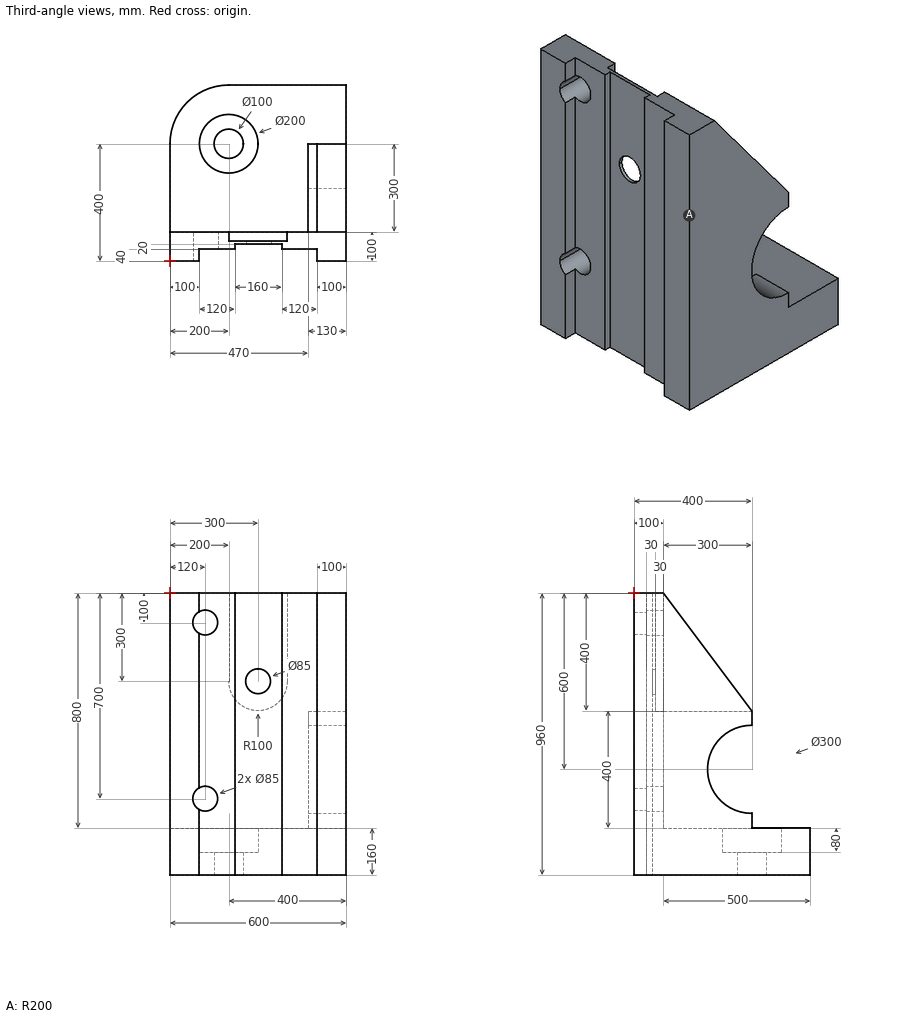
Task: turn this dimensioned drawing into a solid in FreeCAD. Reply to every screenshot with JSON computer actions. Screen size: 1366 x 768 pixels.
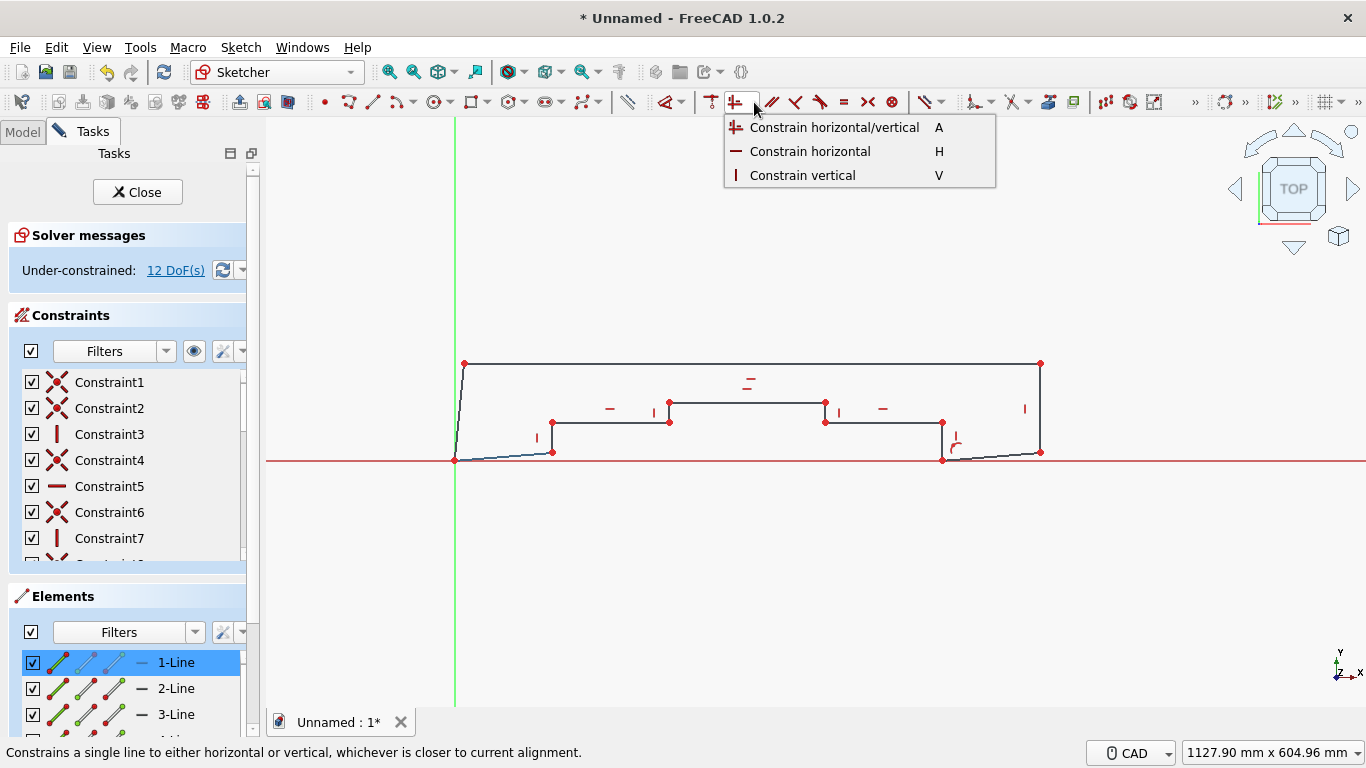
{"action": "left_click", "coordinate": [860, 151]}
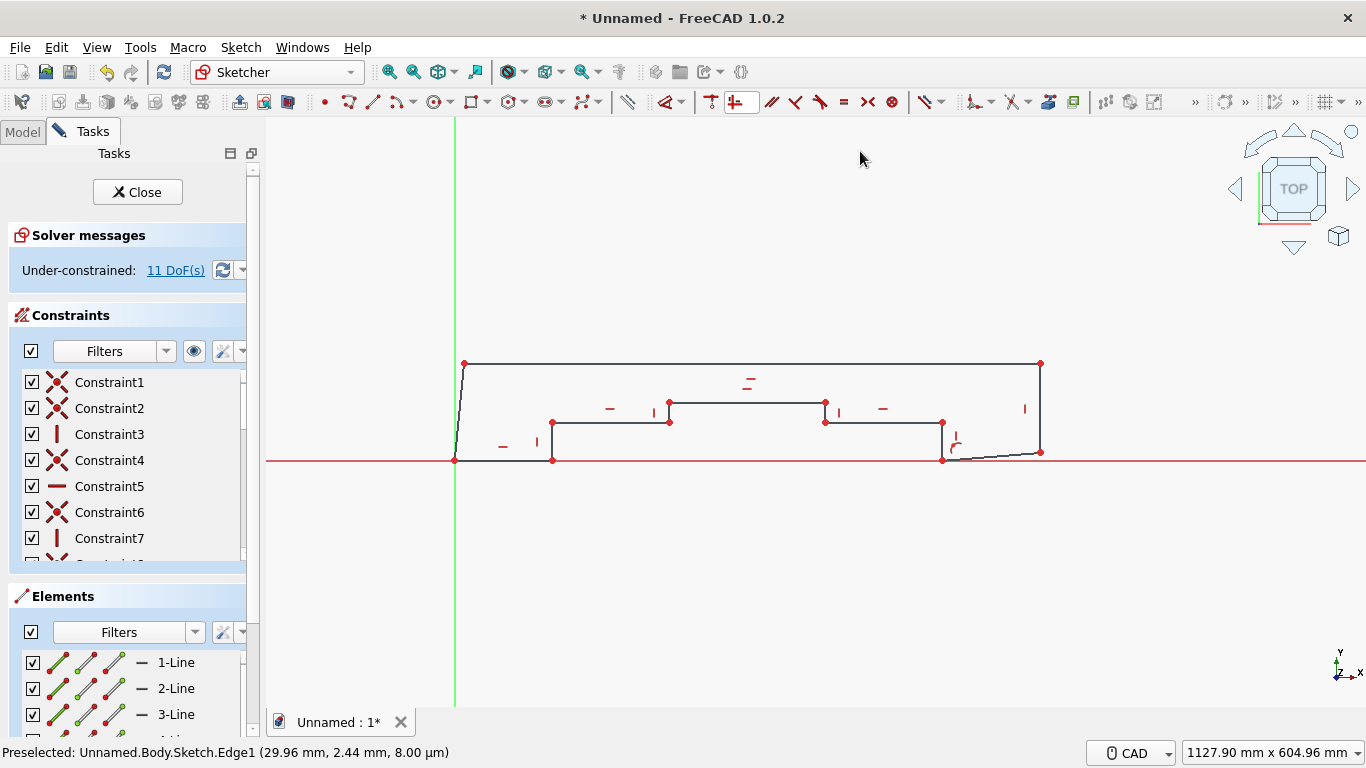
{"action": "left_click", "coordinate": [971, 459]}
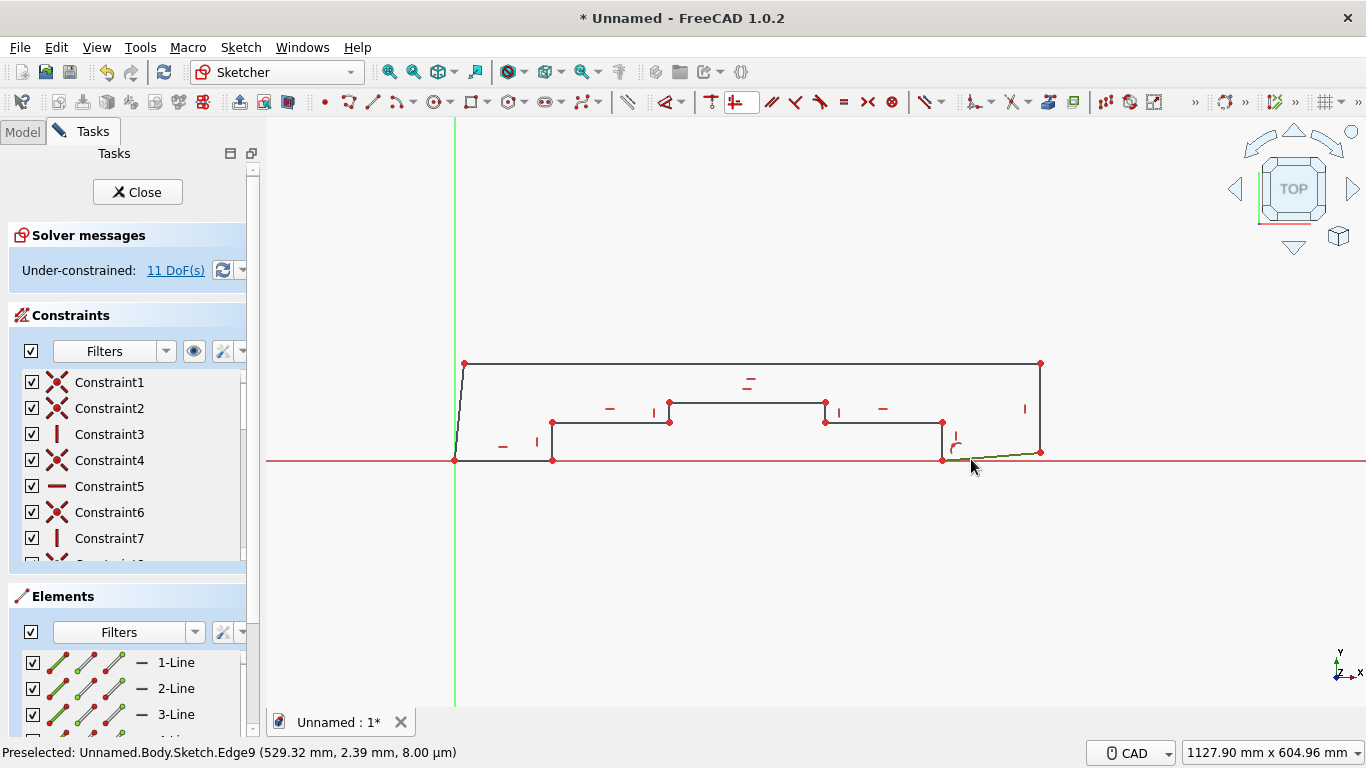
{"action": "key", "text": "h"}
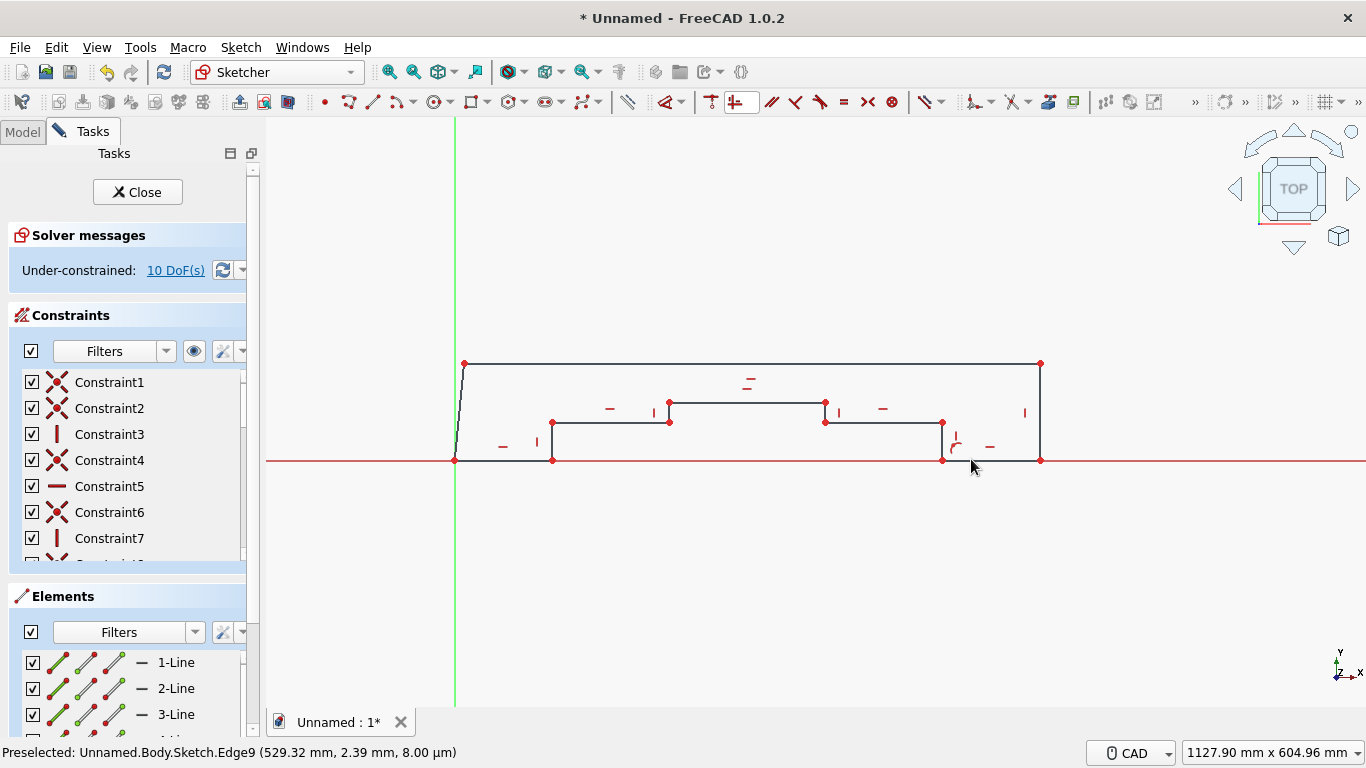
{"action": "left_click", "coordinate": [457, 432]}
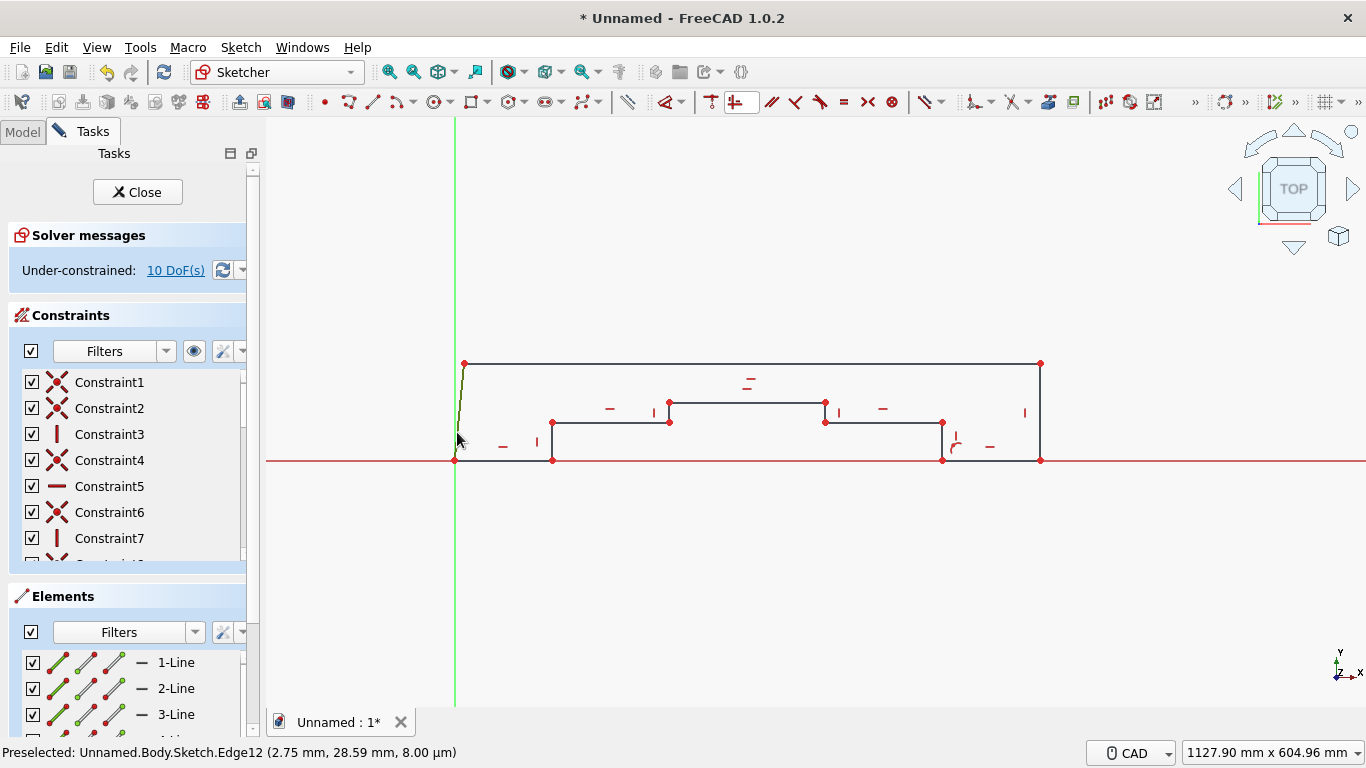
{"action": "key", "text": "v"}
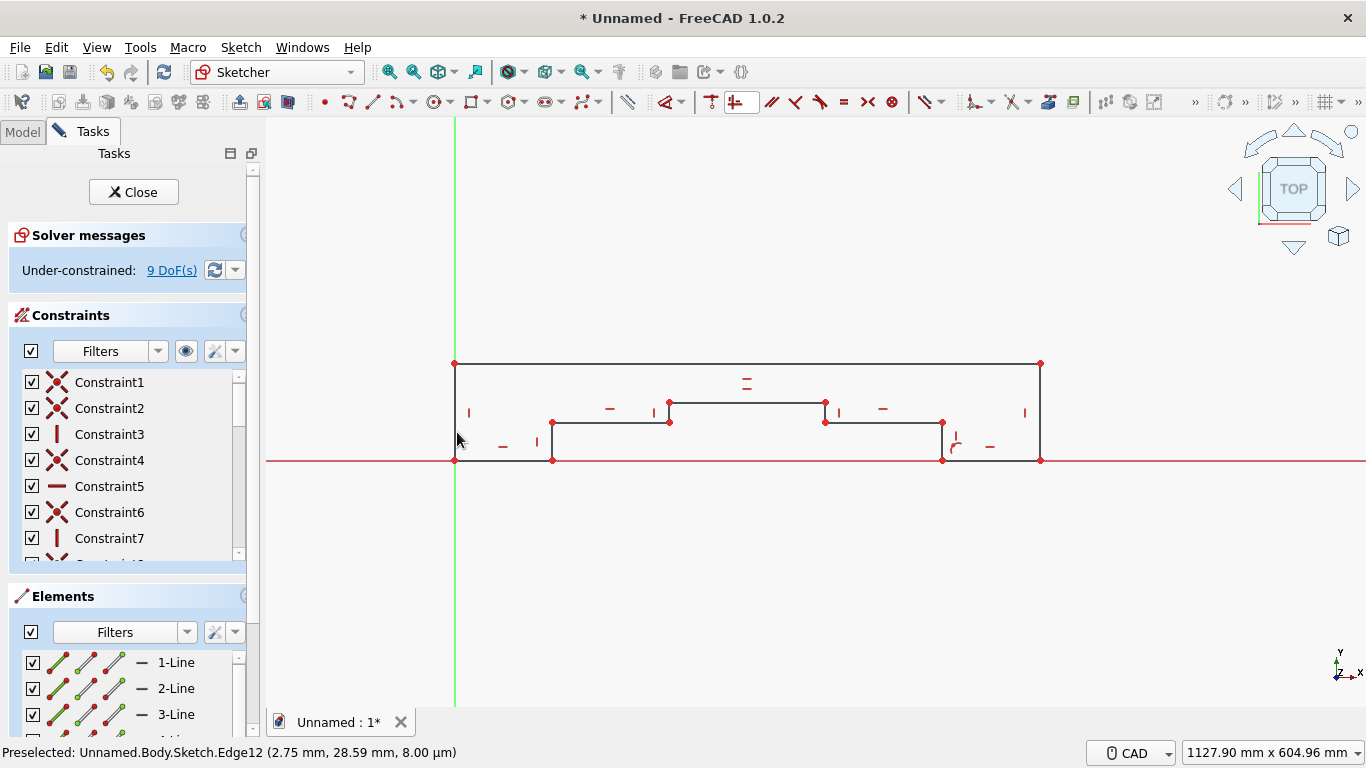
{"action": "left_click", "coordinate": [552, 450]}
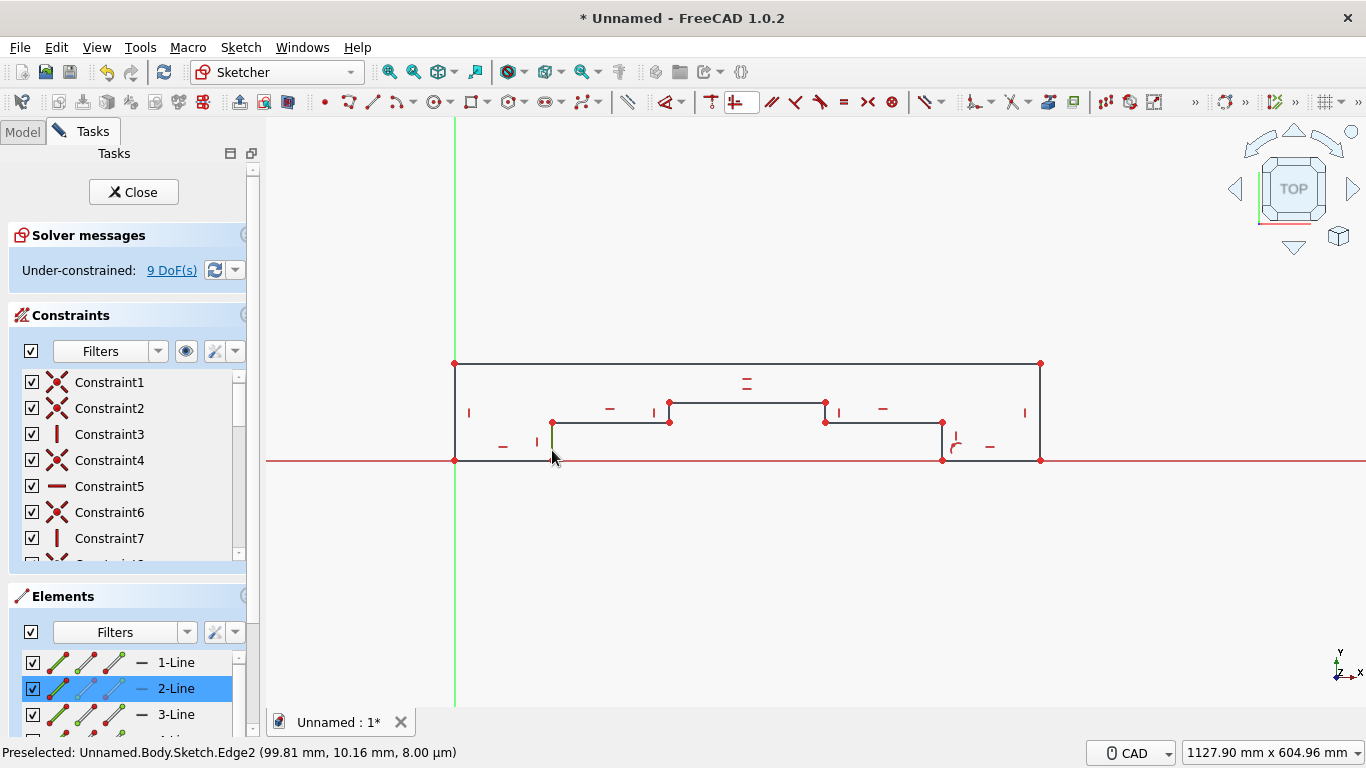
{"action": "left_click", "coordinate": [684, 102]}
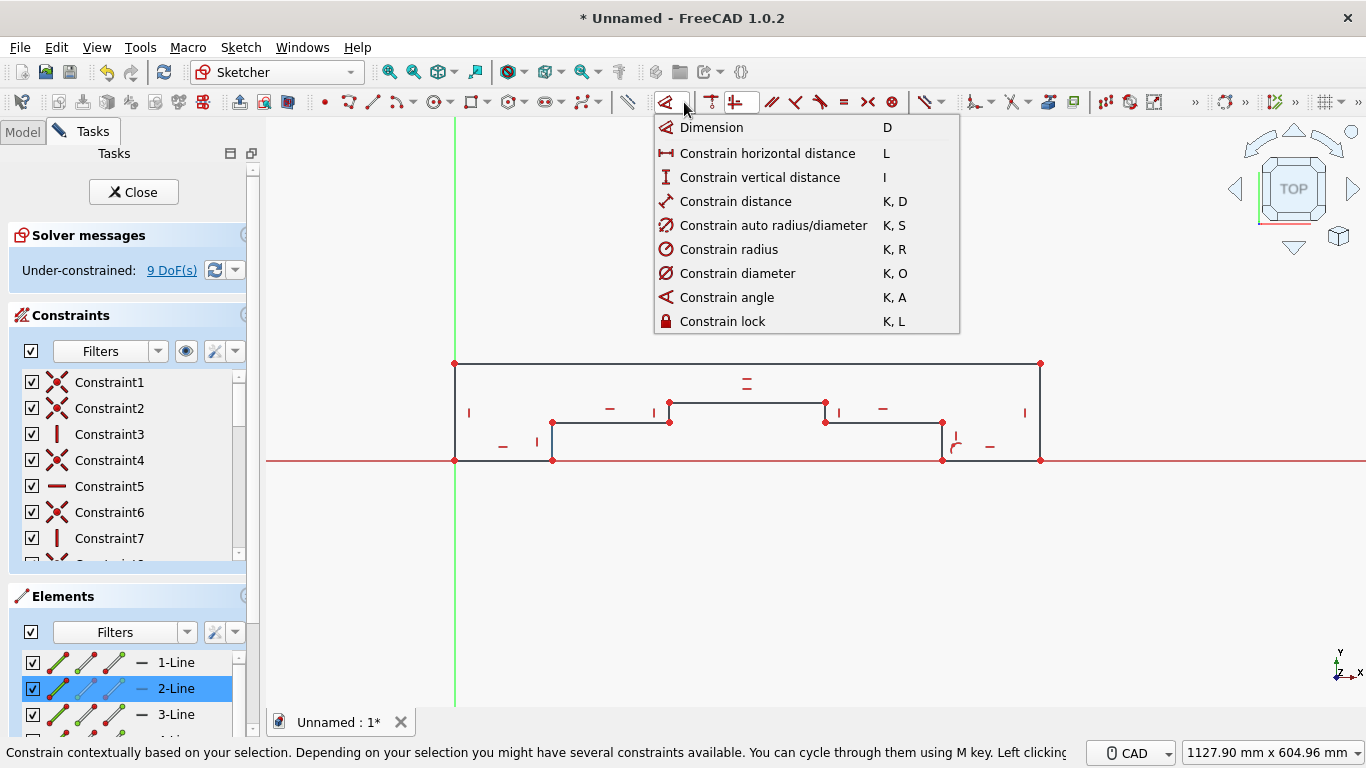
{"action": "left_click", "coordinate": [807, 177]}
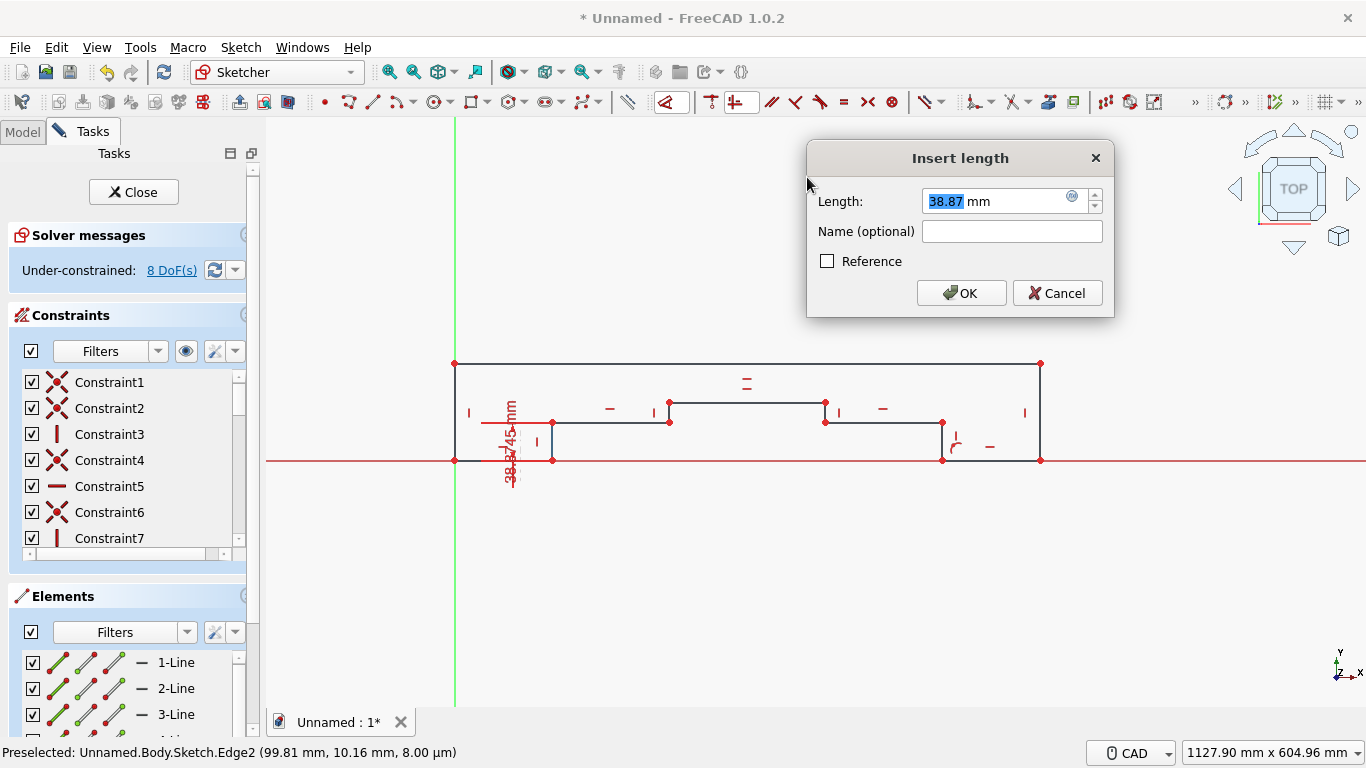
{"action": "type", "text": "40"}
{"action": "key", "text": "Return"}